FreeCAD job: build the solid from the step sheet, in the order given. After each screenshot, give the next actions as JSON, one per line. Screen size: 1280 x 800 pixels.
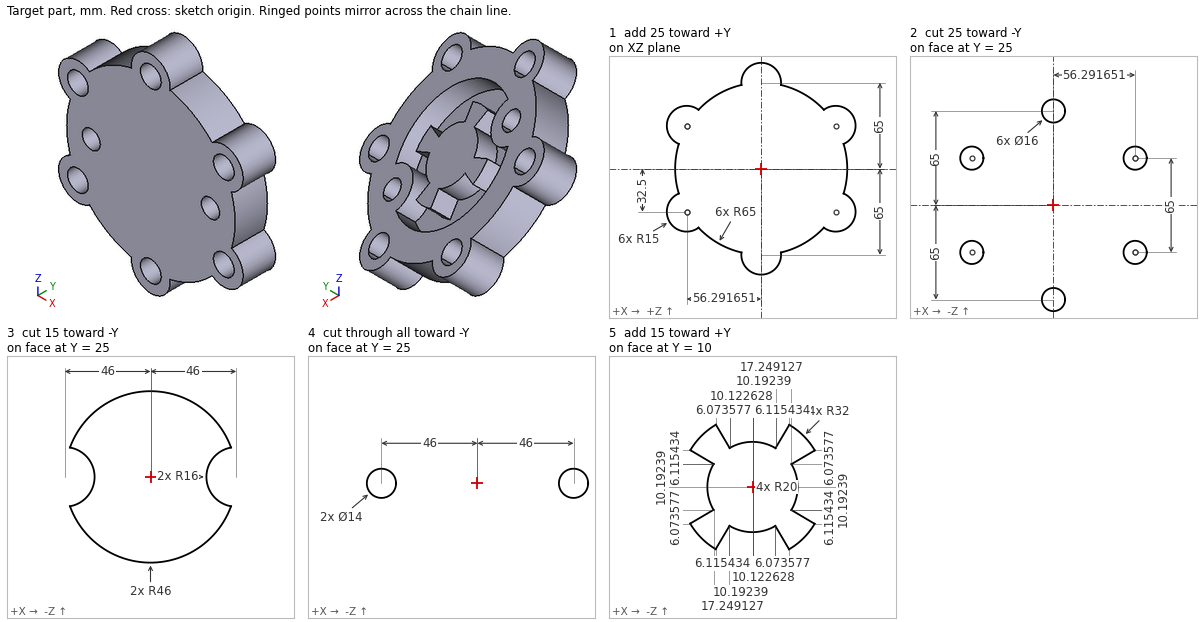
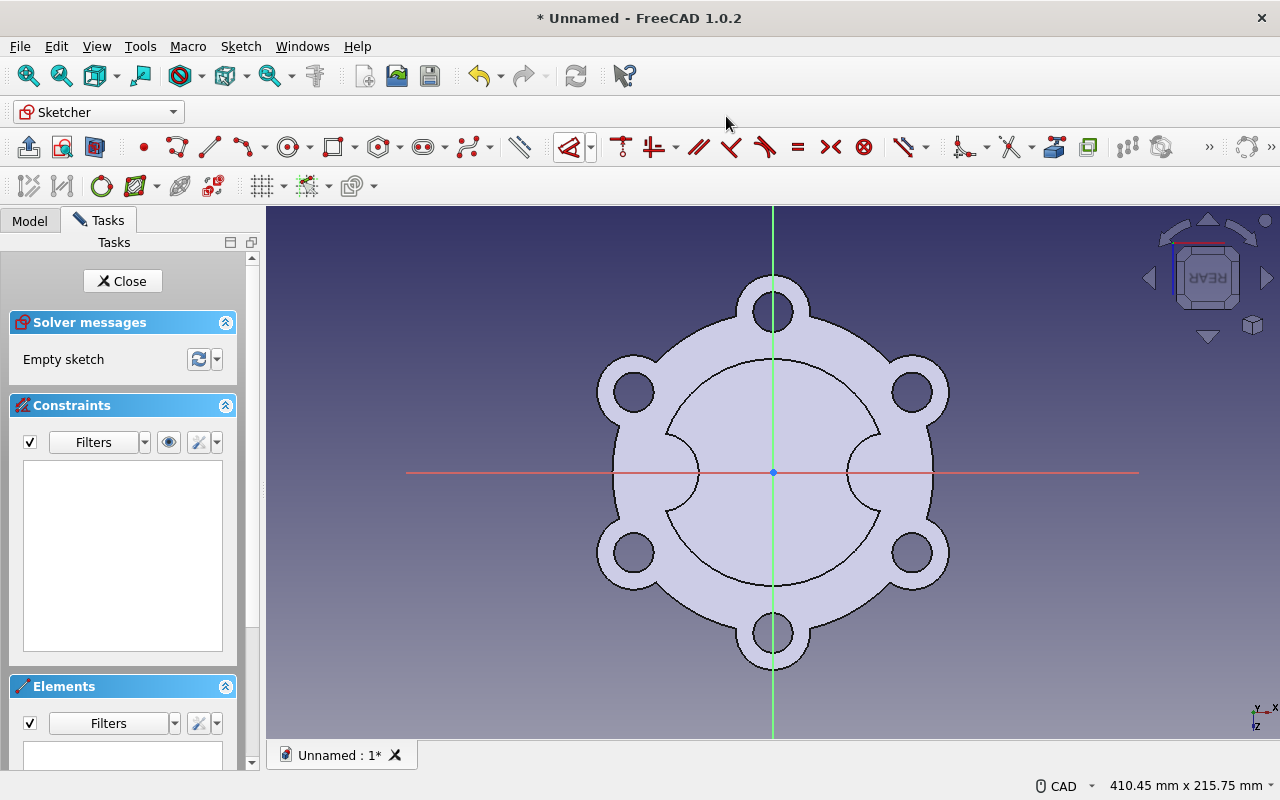
{"action": "scroll", "coordinate": [829, 472], "scroll_direction": "up", "scroll_amount": 4}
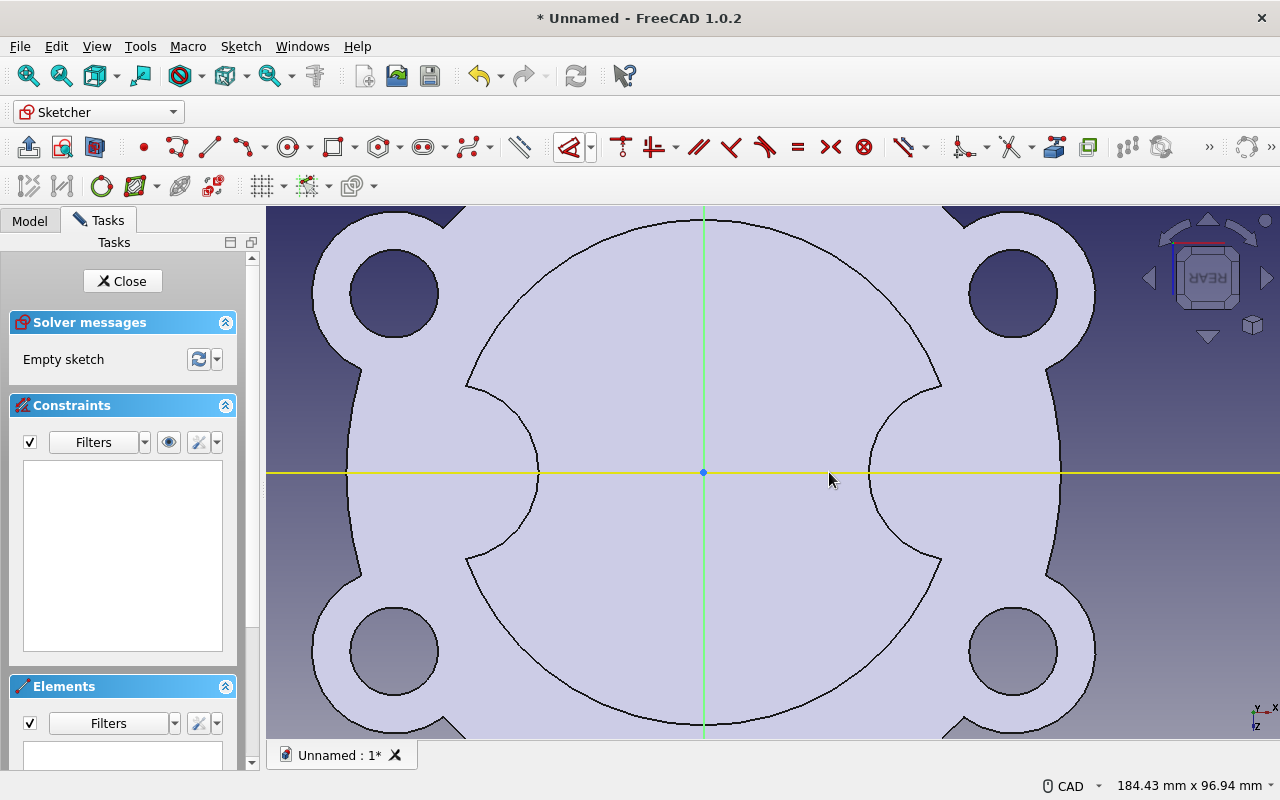
{"action": "left_click", "coordinate": [288, 148]}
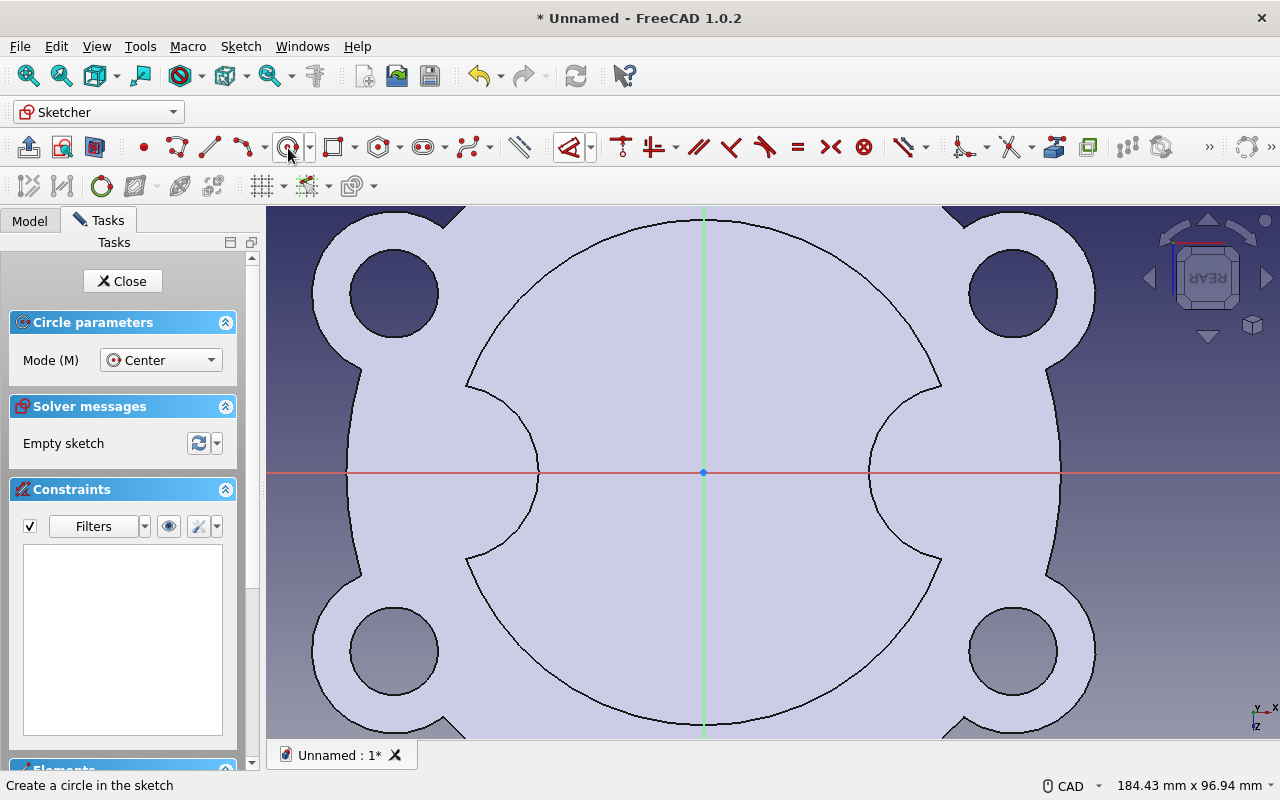
{"action": "left_click", "coordinate": [451, 472]}
{"action": "mouse_move", "coordinate": [478, 445]}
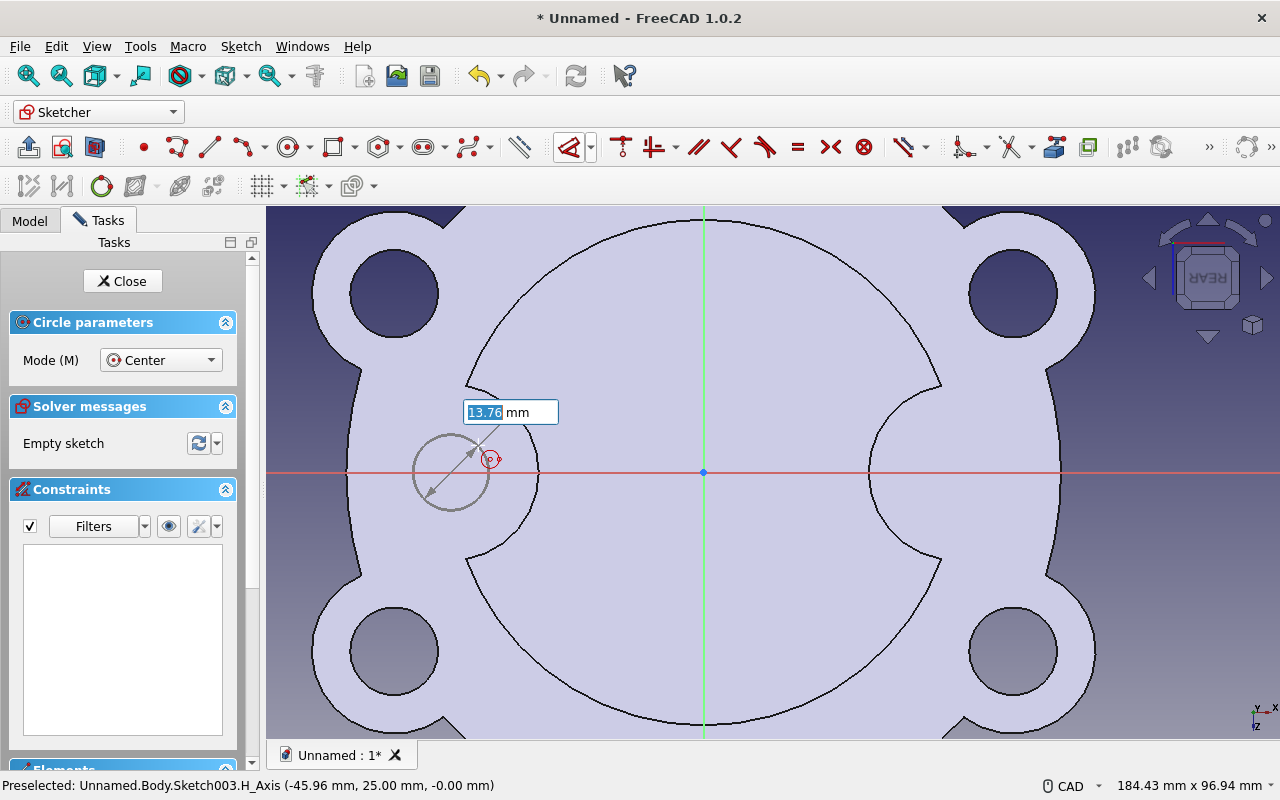
{"action": "type", "text": "14"}
{"action": "key", "text": "Return"}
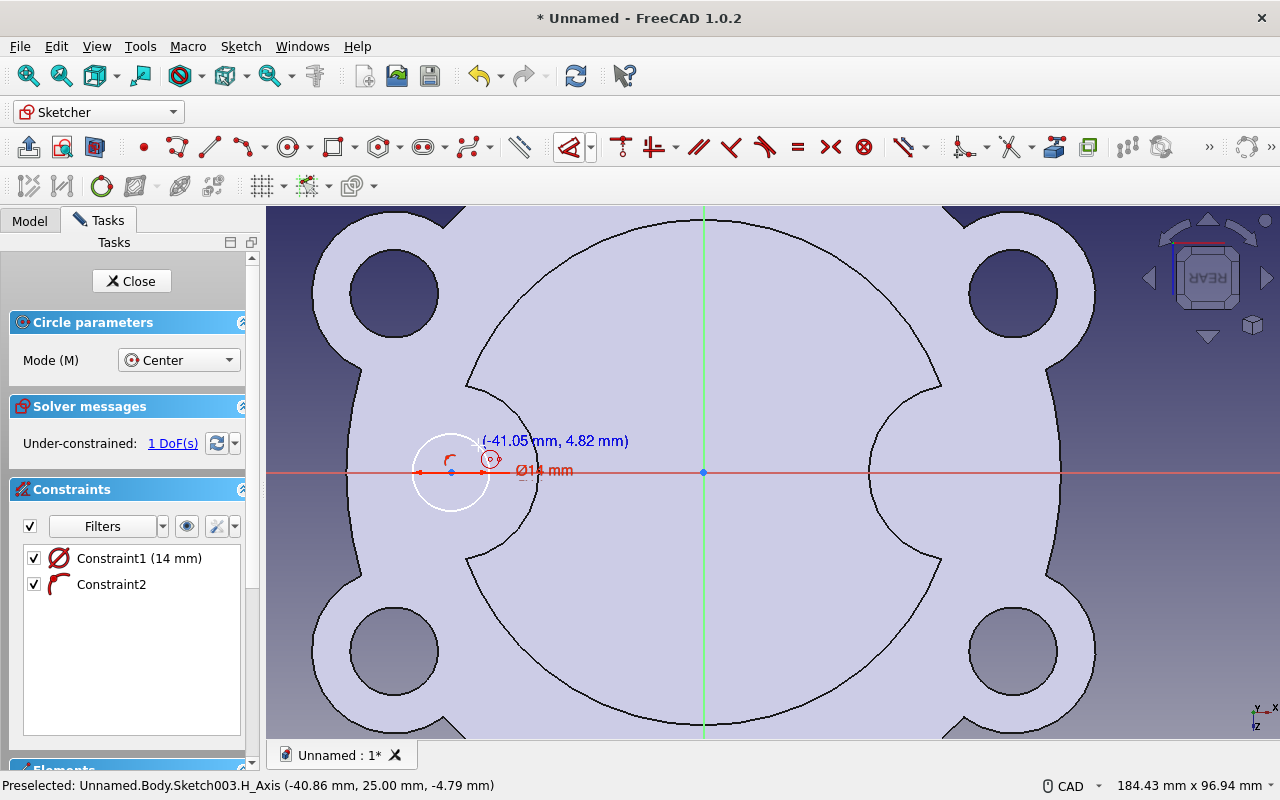
{"action": "left_click", "coordinate": [957, 472]}
{"action": "mouse_move", "coordinate": [984, 445]}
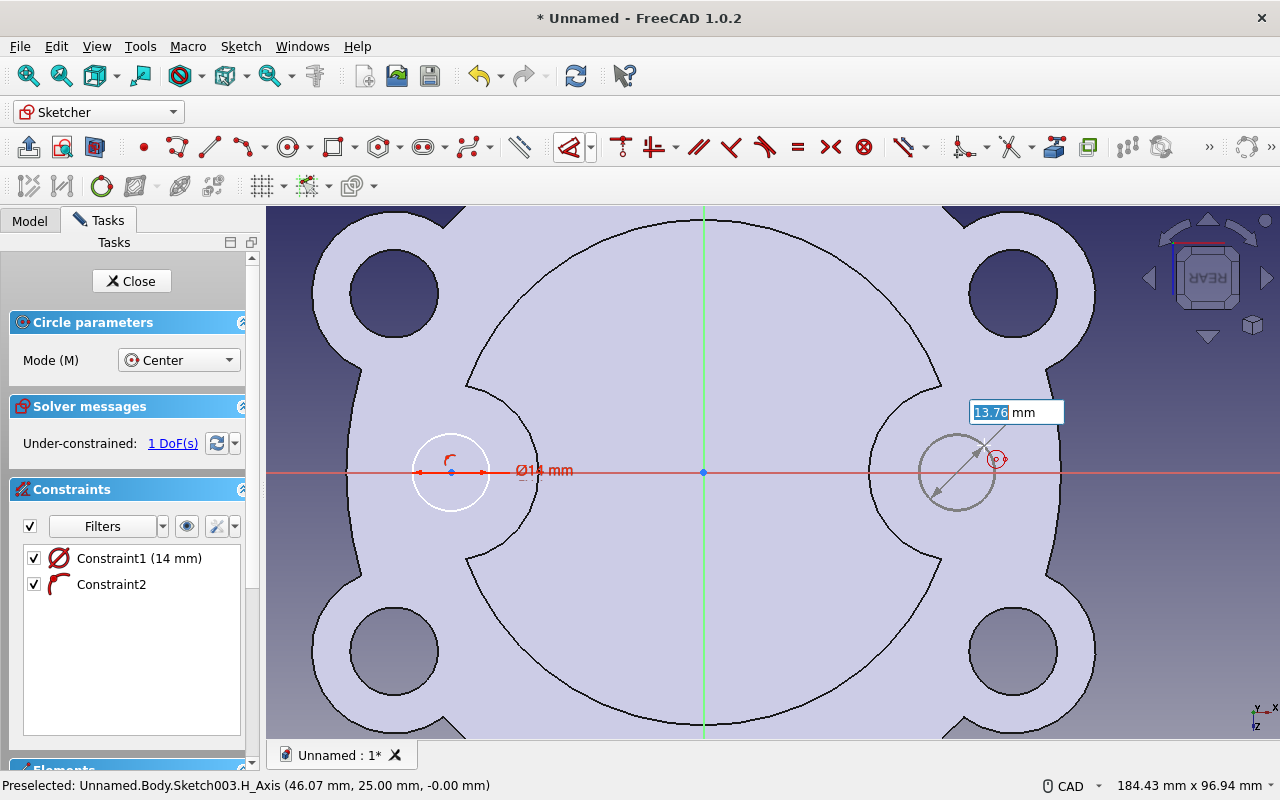
{"action": "type", "text": "14"}
{"action": "key", "text": "Return"}
{"action": "key", "text": "Escape"}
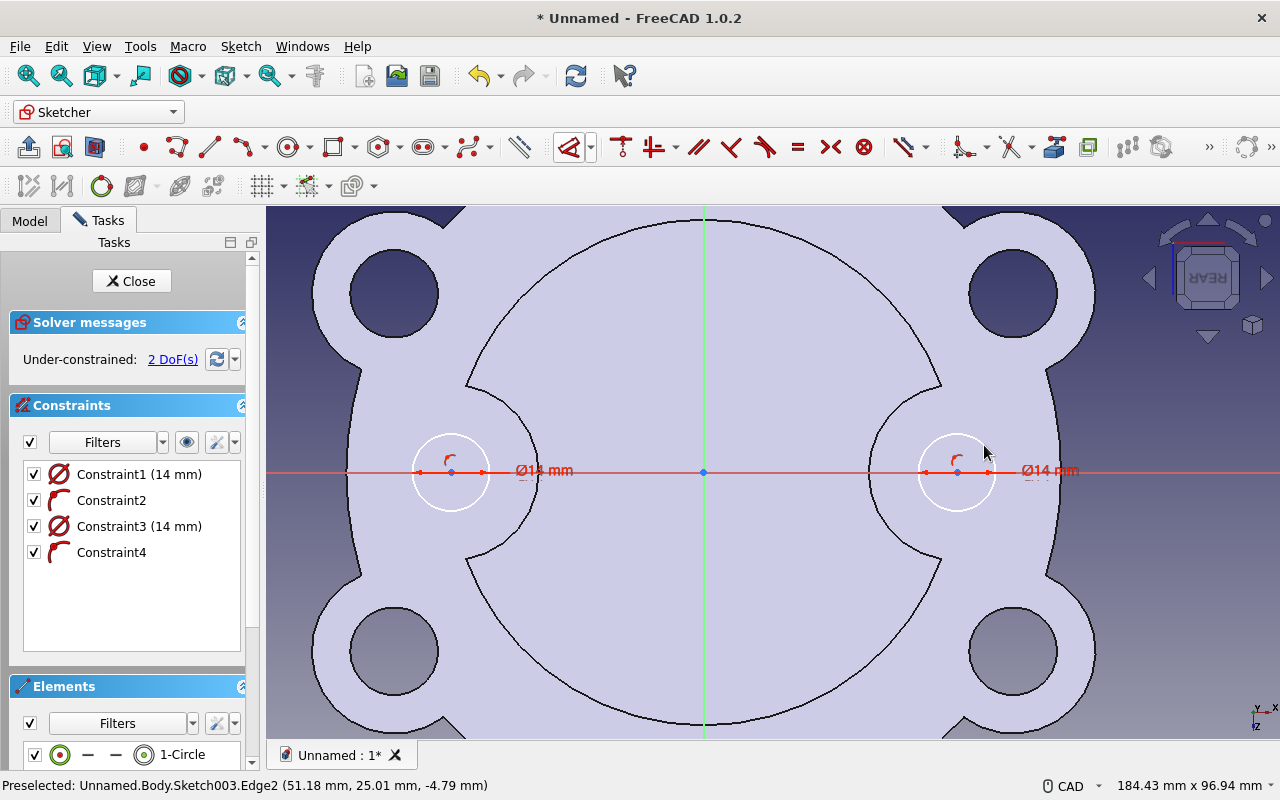
{"action": "left_click", "coordinate": [451, 472]}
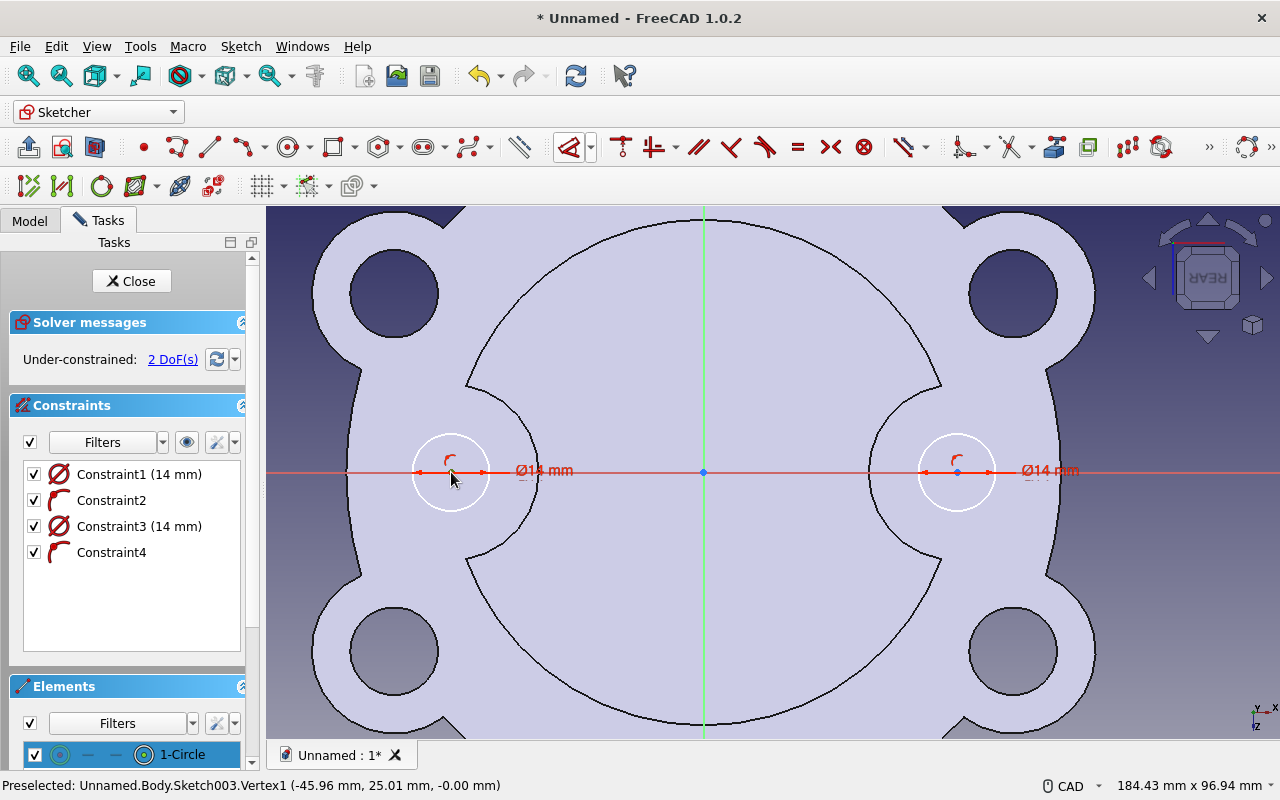
{"action": "key", "text": "l"}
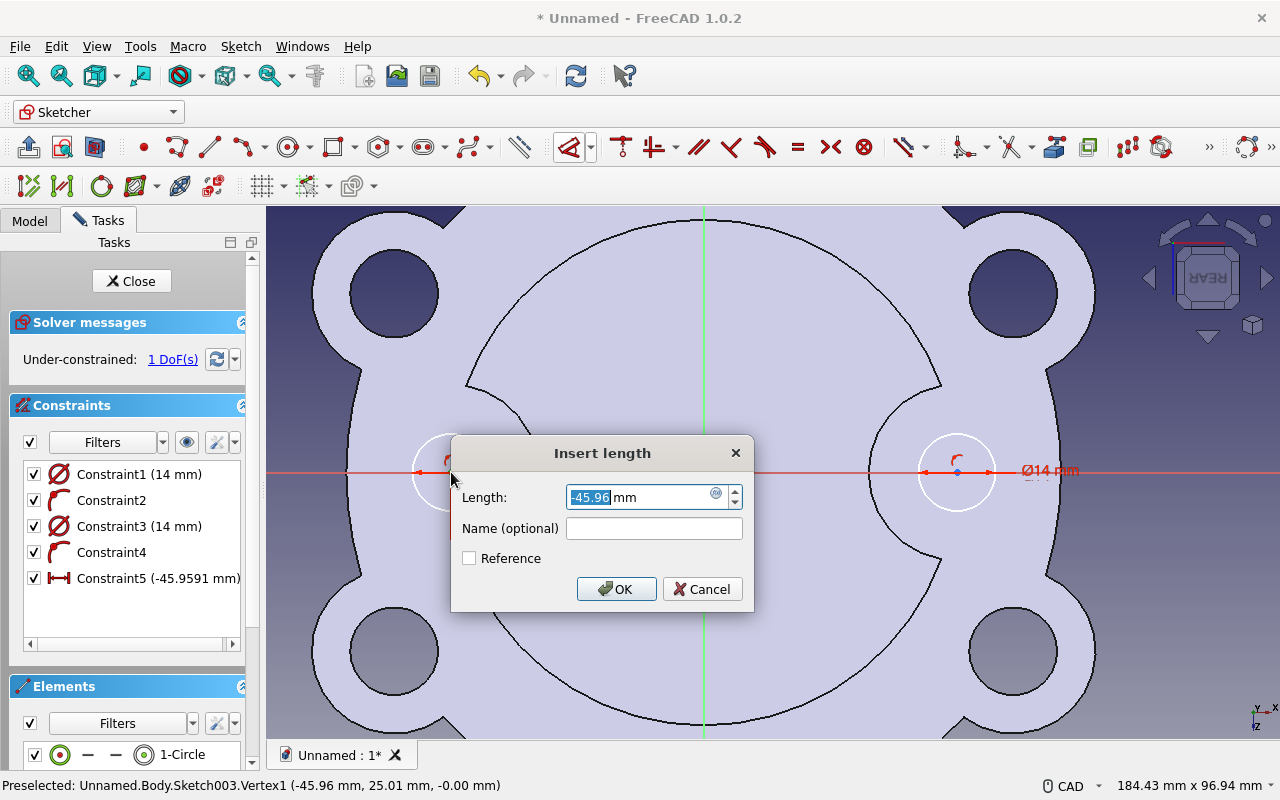
{"action": "type", "text": "-46"}
{"action": "key", "text": "Return"}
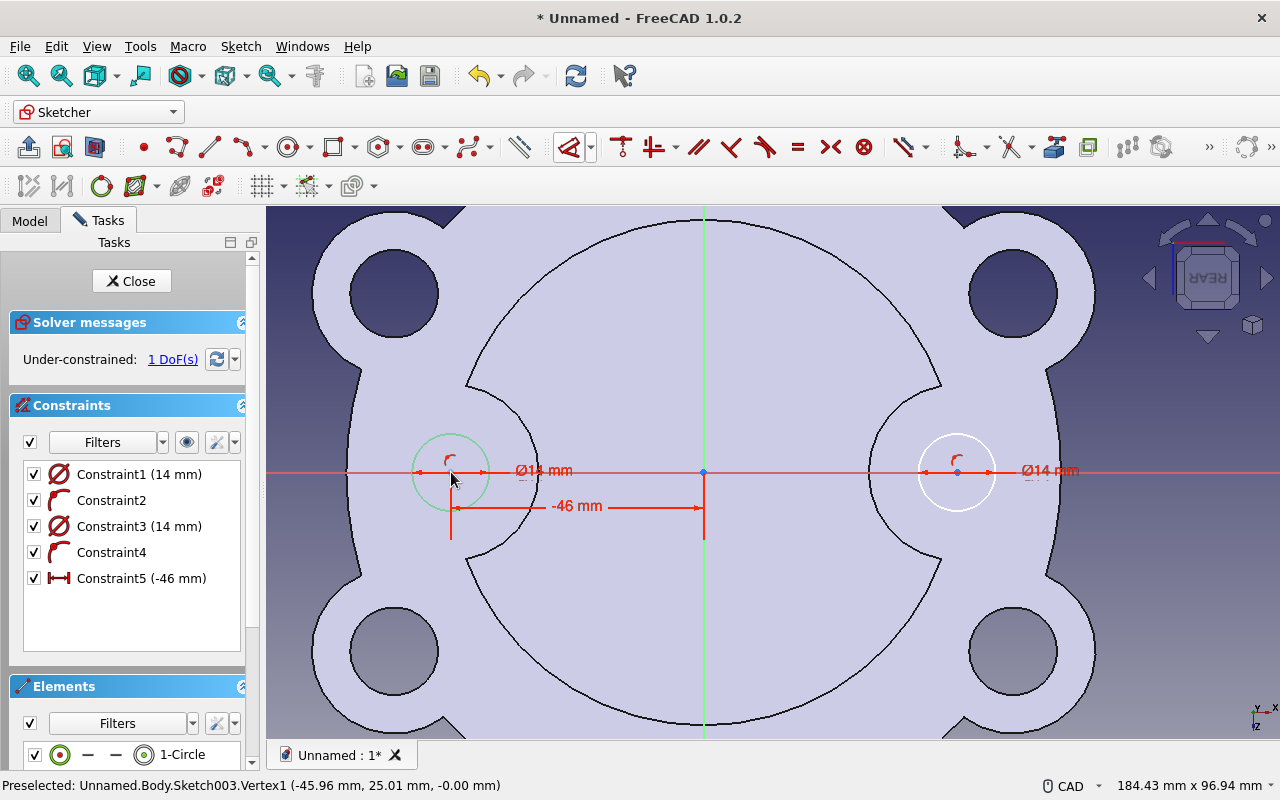
{"action": "left_click", "coordinate": [957, 472]}